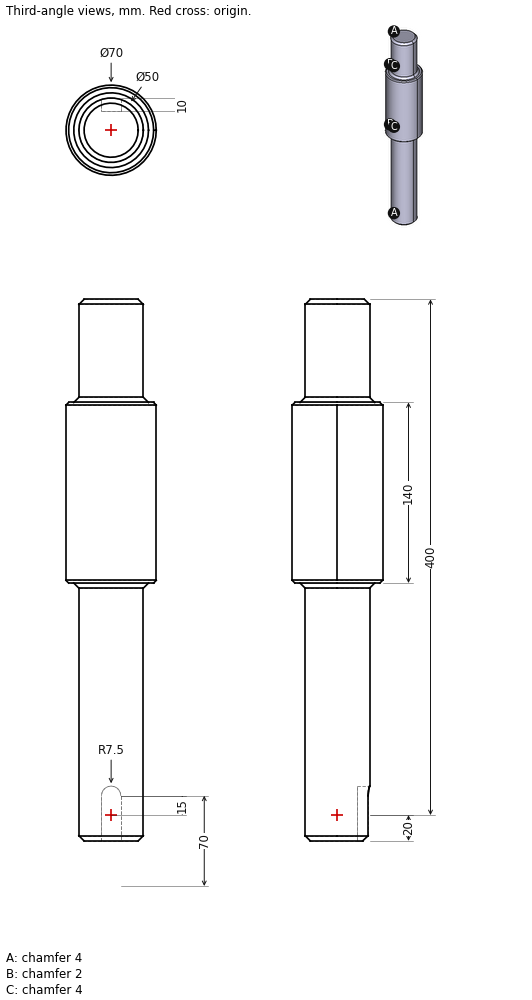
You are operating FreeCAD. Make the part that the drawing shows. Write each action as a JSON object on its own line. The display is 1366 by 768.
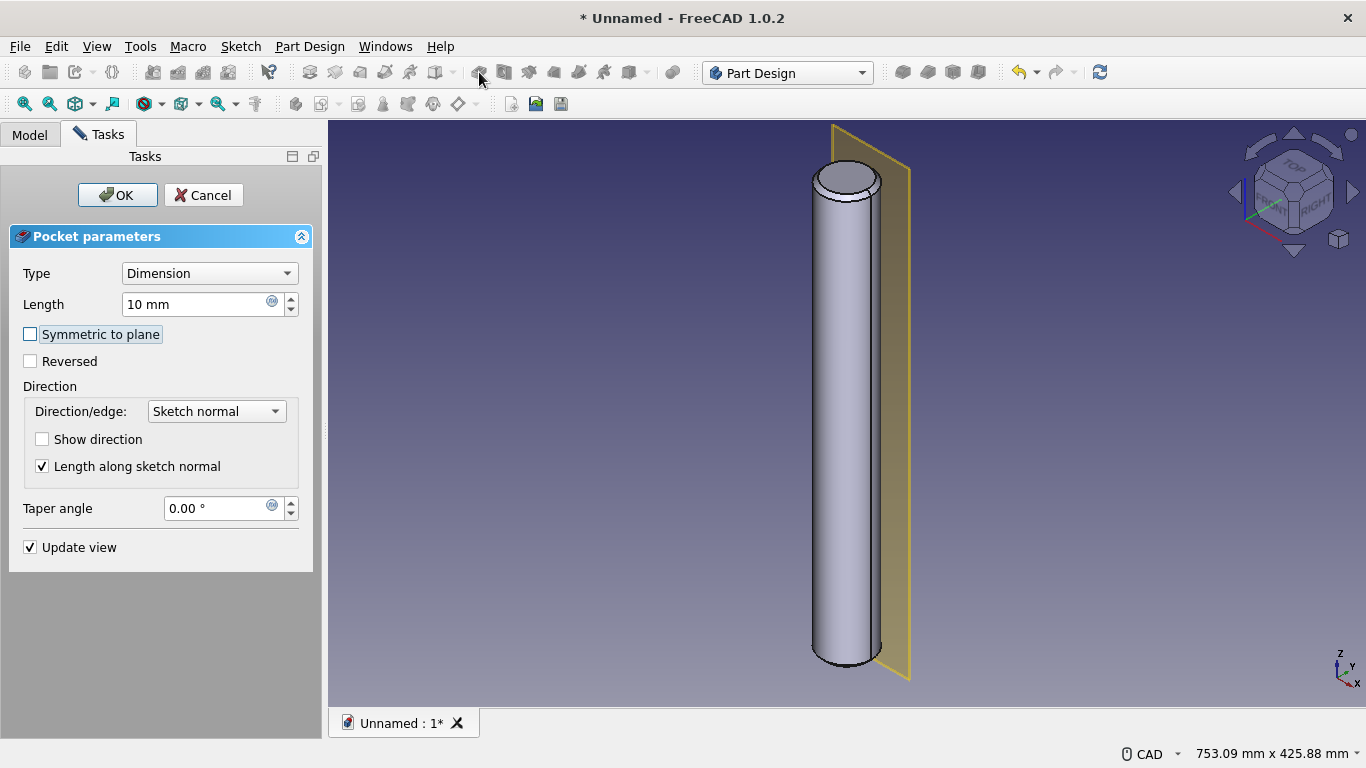
{"action": "left_click", "coordinate": [31, 361]}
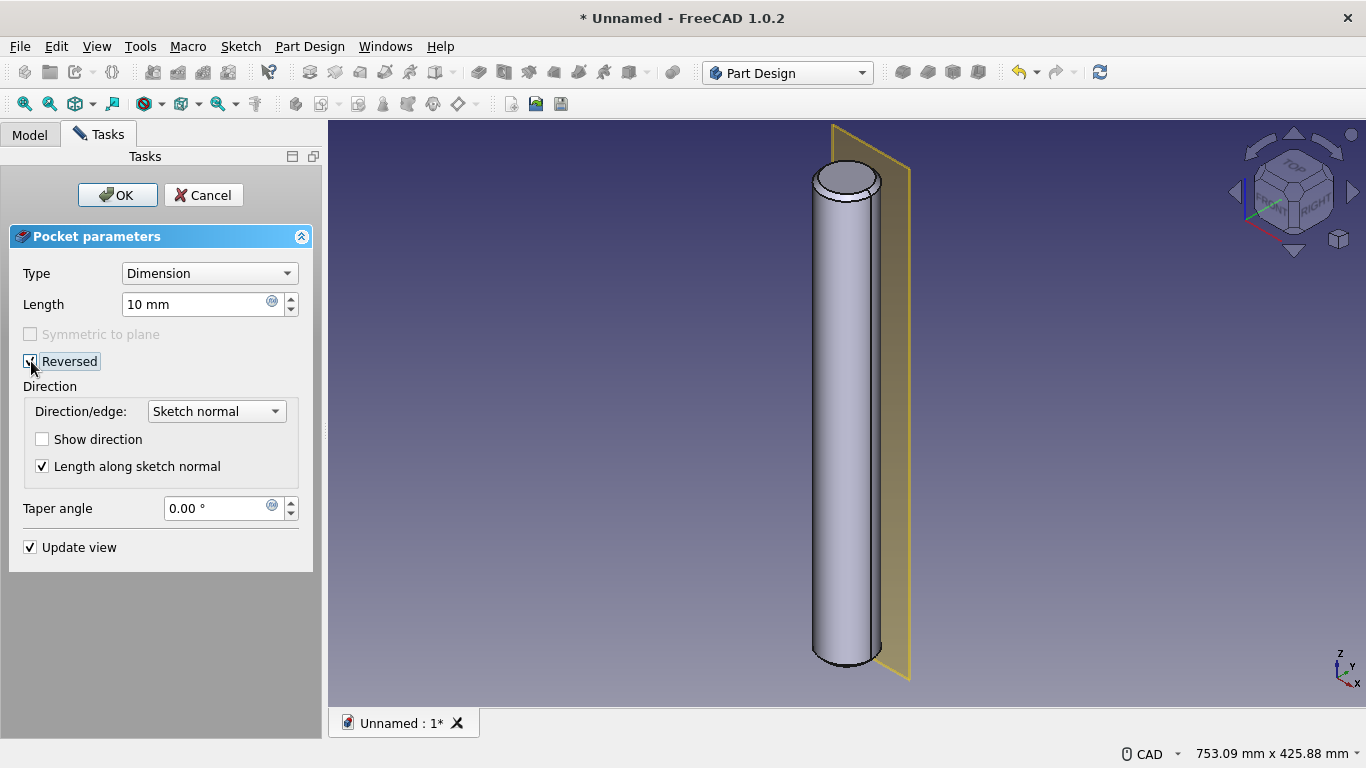
{"action": "left_click", "coordinate": [118, 195]}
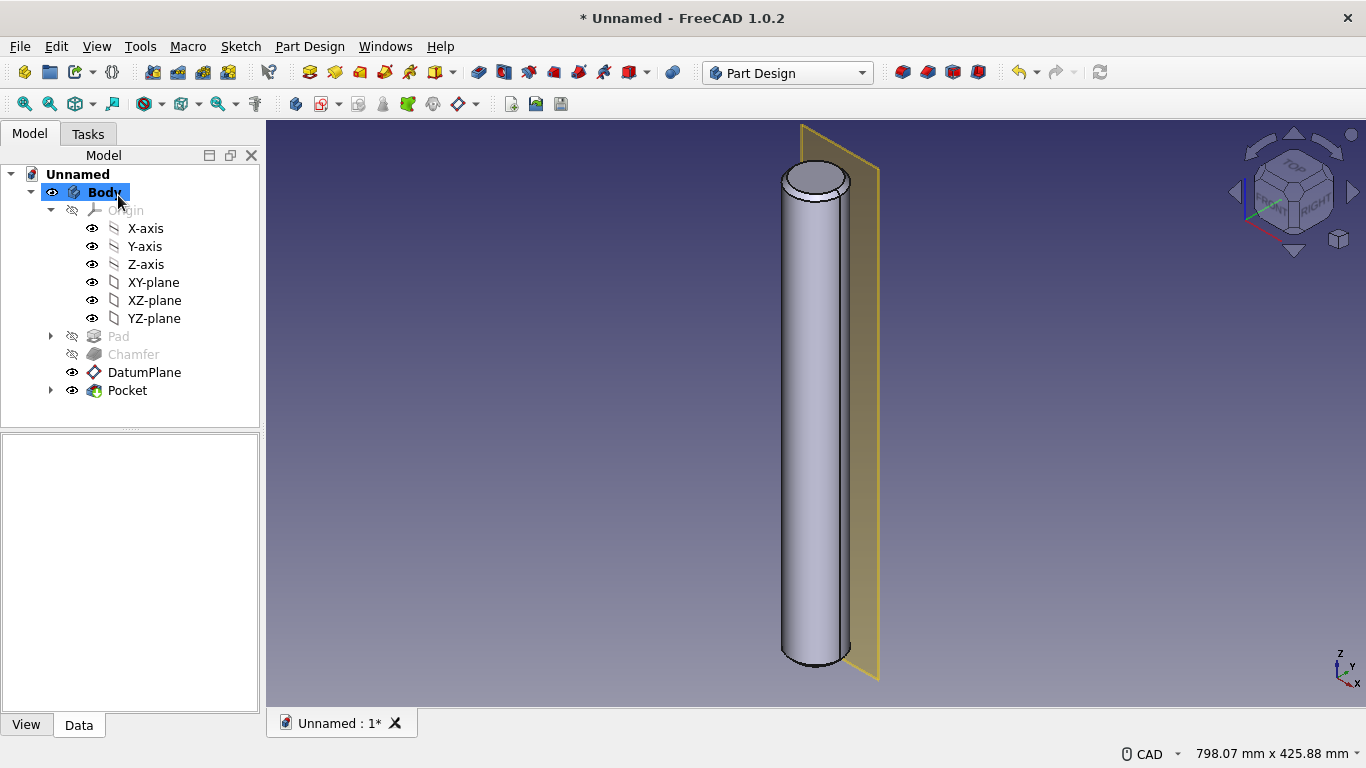
{"action": "left_click", "coordinate": [117, 372]}
{"action": "key", "text": "space"}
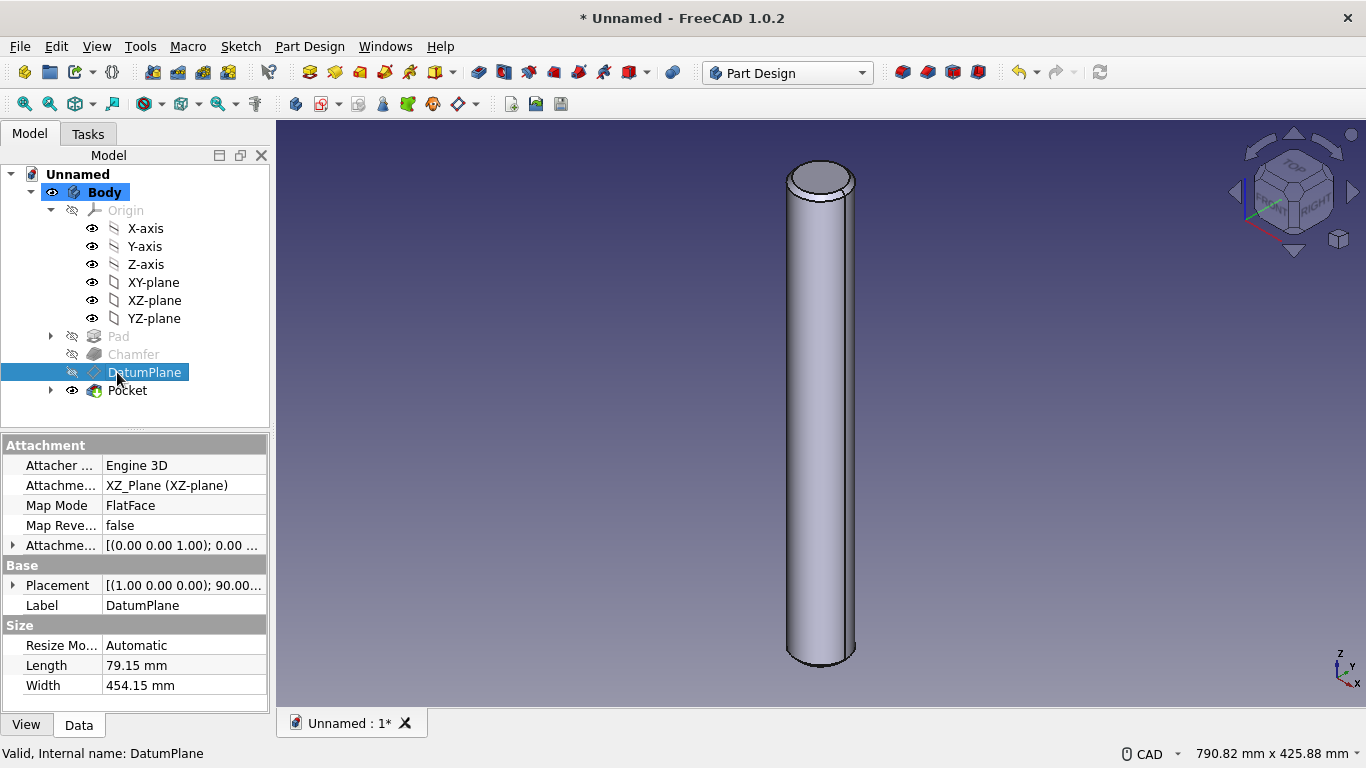
{"action": "left_click", "coordinate": [137, 282]}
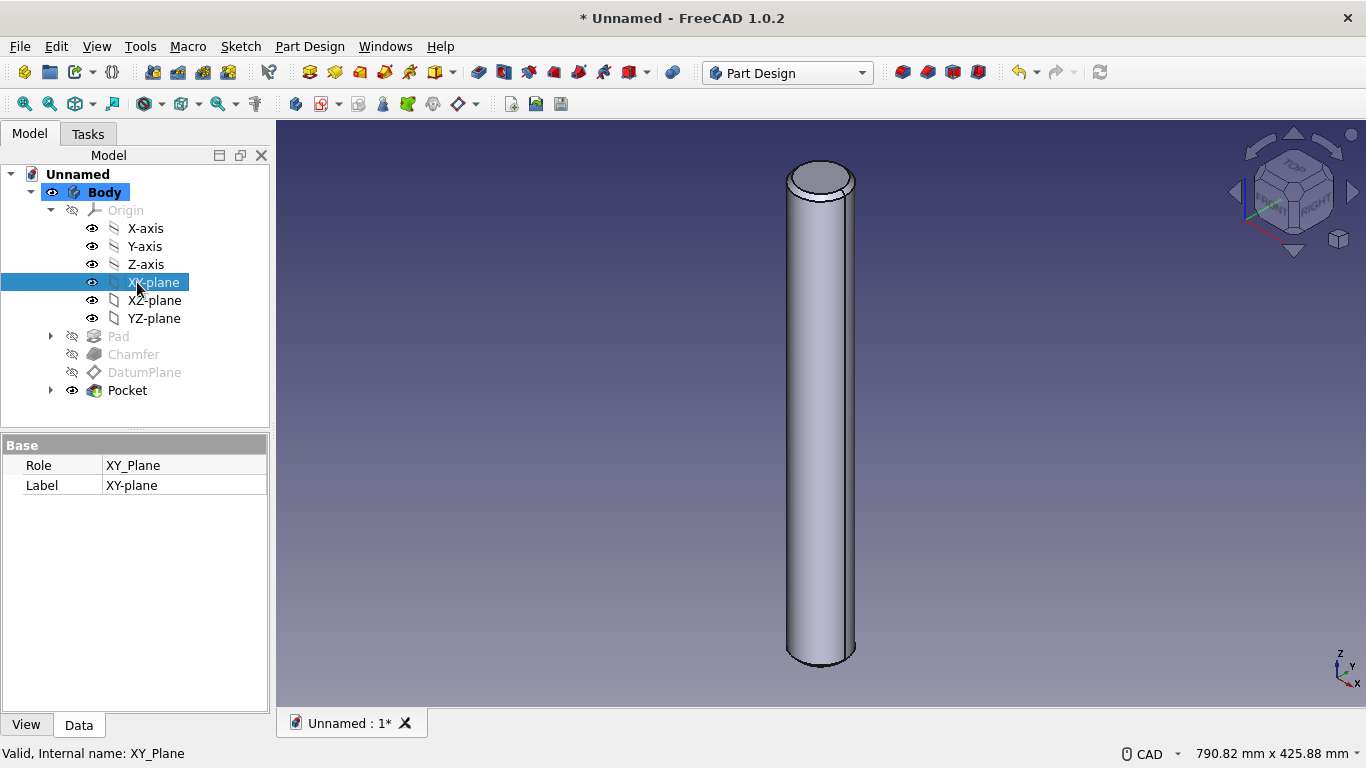
{"action": "left_click", "coordinate": [458, 104]}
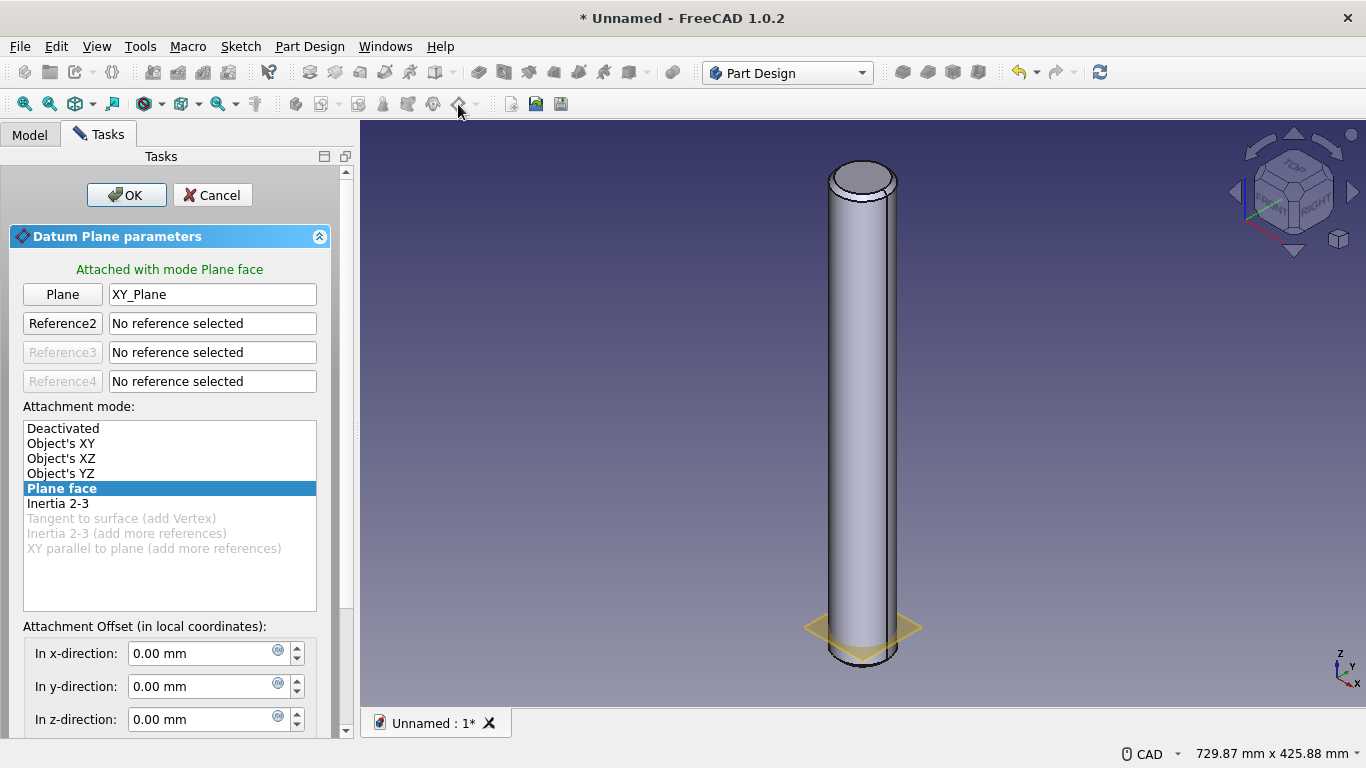
{"action": "triple_click", "coordinate": [210, 720]}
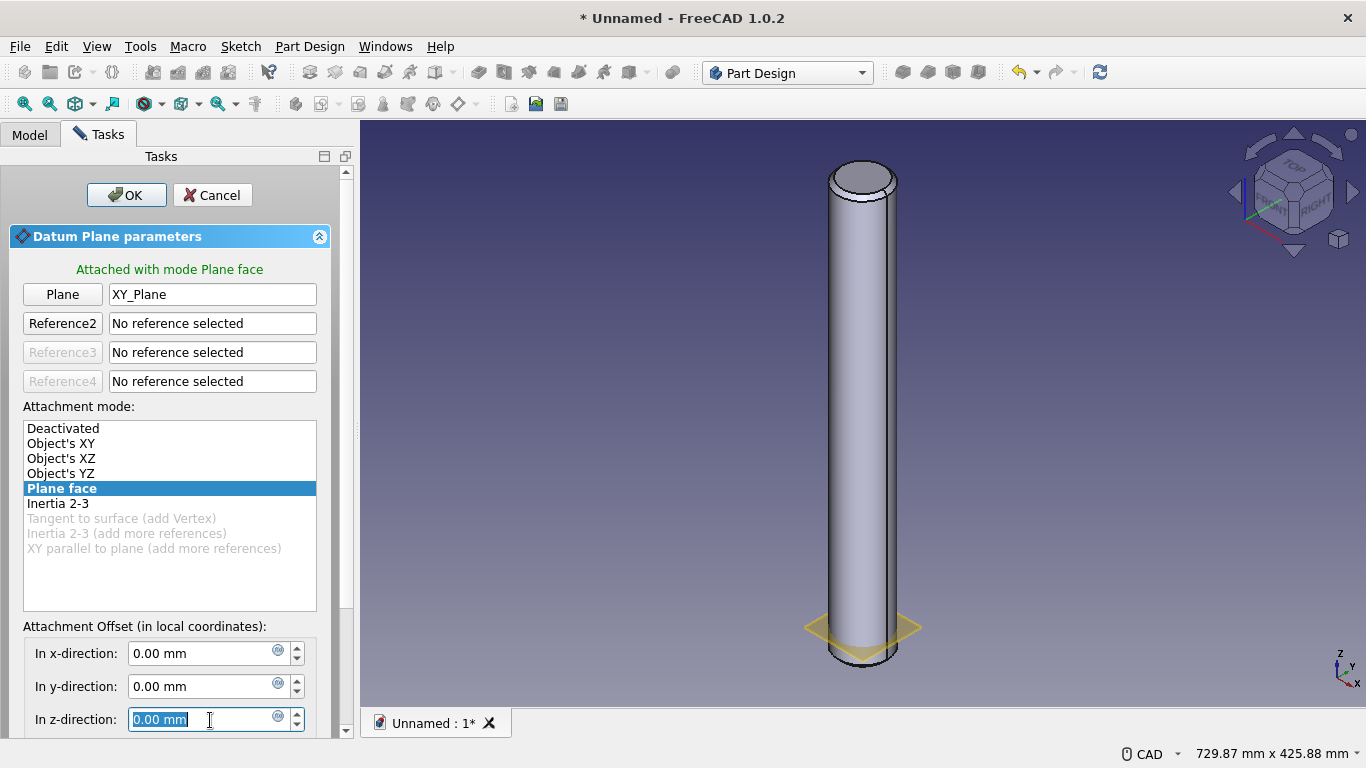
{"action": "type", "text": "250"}
{"action": "key", "text": "Tab"}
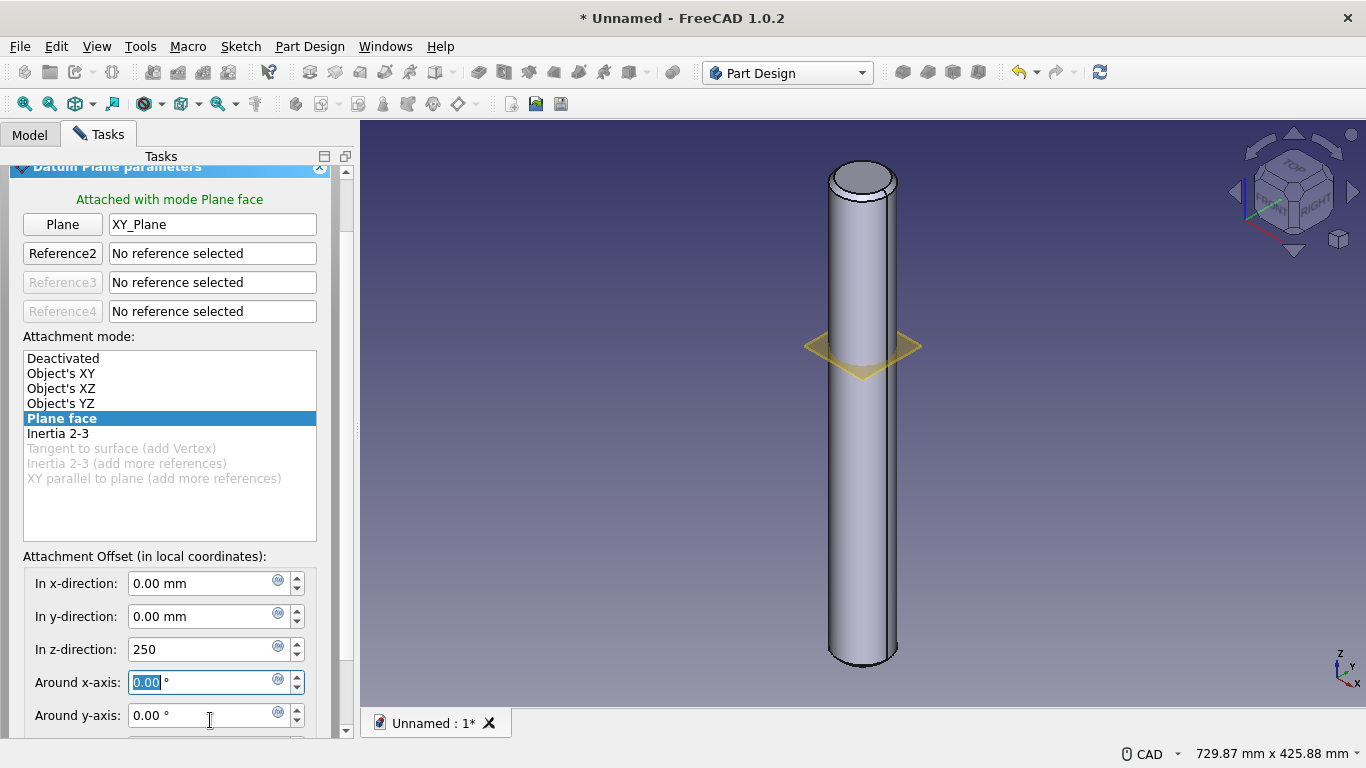
{"action": "scroll", "coordinate": [346, 452], "scroll_direction": "up", "scroll_amount": 2}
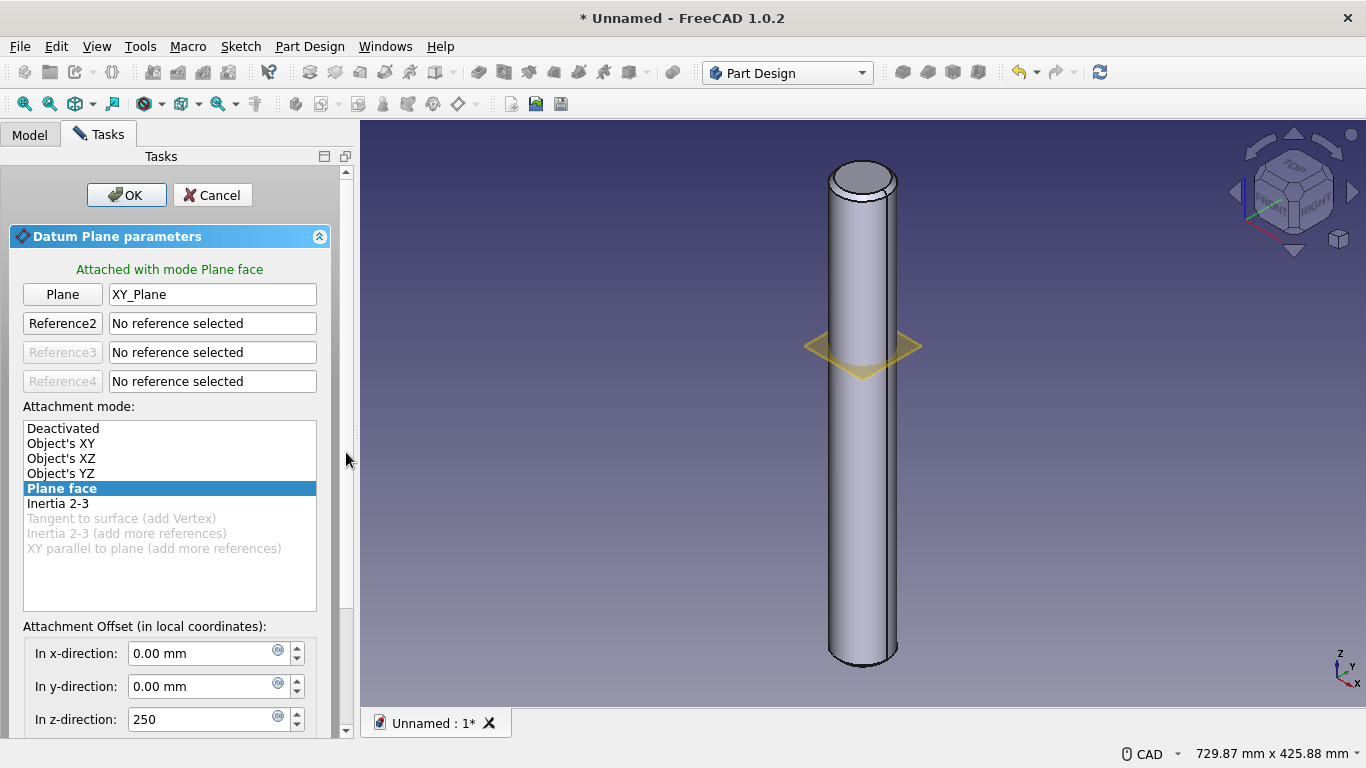
{"action": "left_click", "coordinate": [127, 195]}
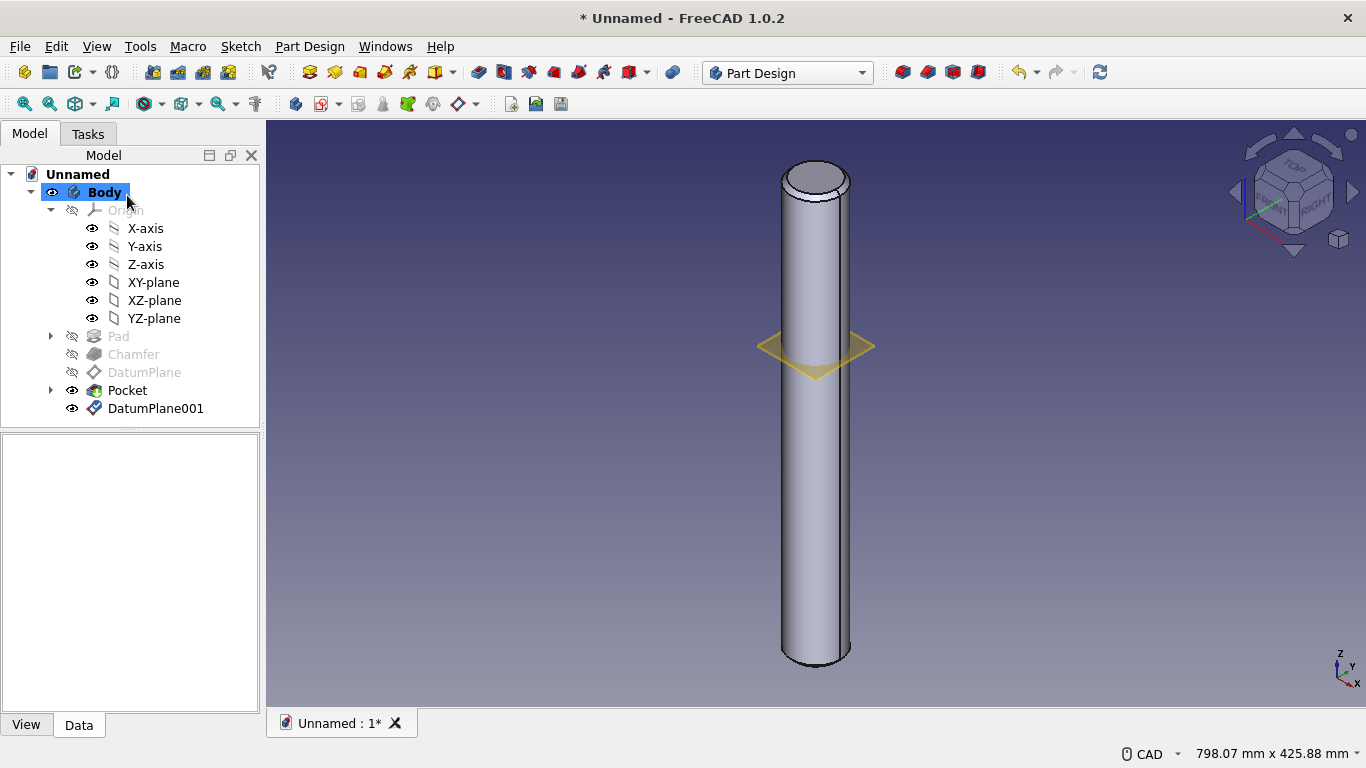
{"action": "left_click", "coordinate": [117, 408]}